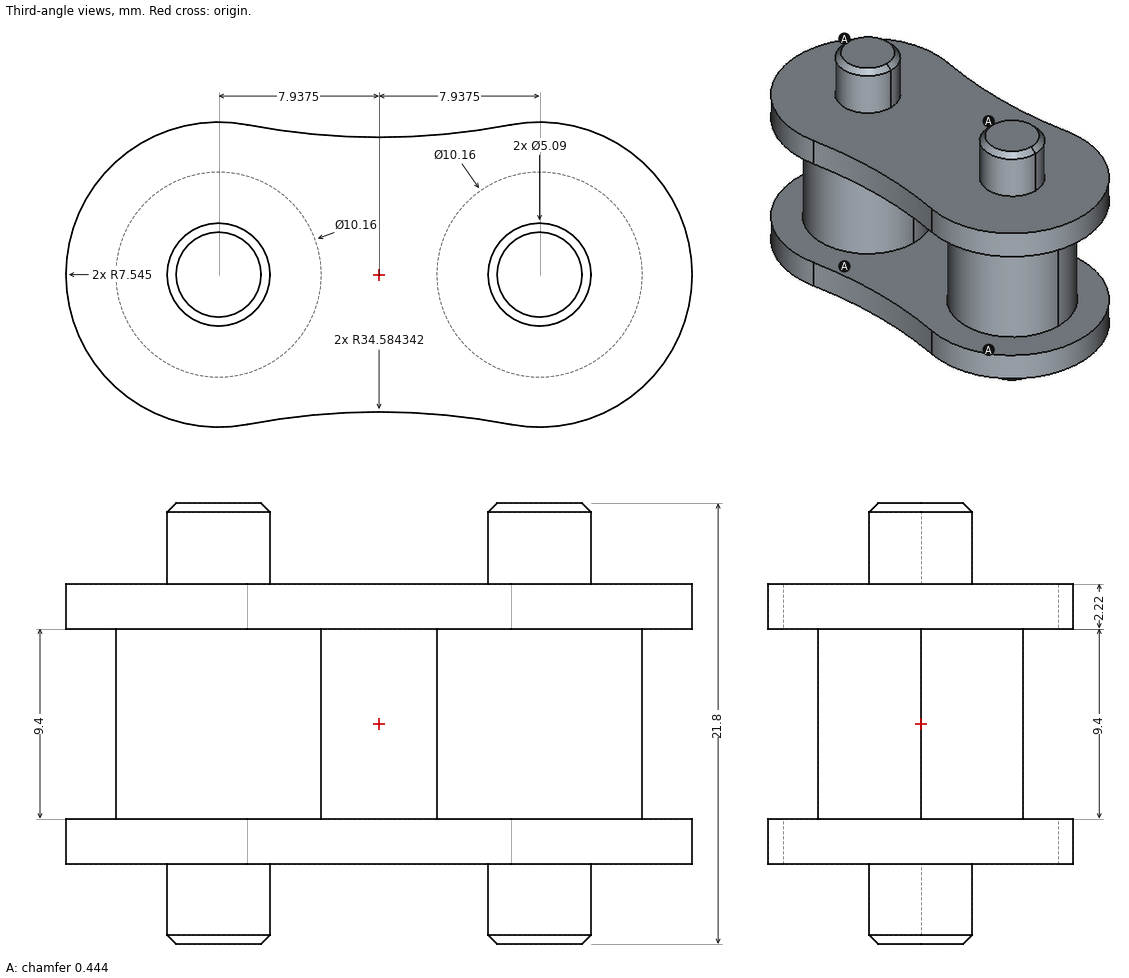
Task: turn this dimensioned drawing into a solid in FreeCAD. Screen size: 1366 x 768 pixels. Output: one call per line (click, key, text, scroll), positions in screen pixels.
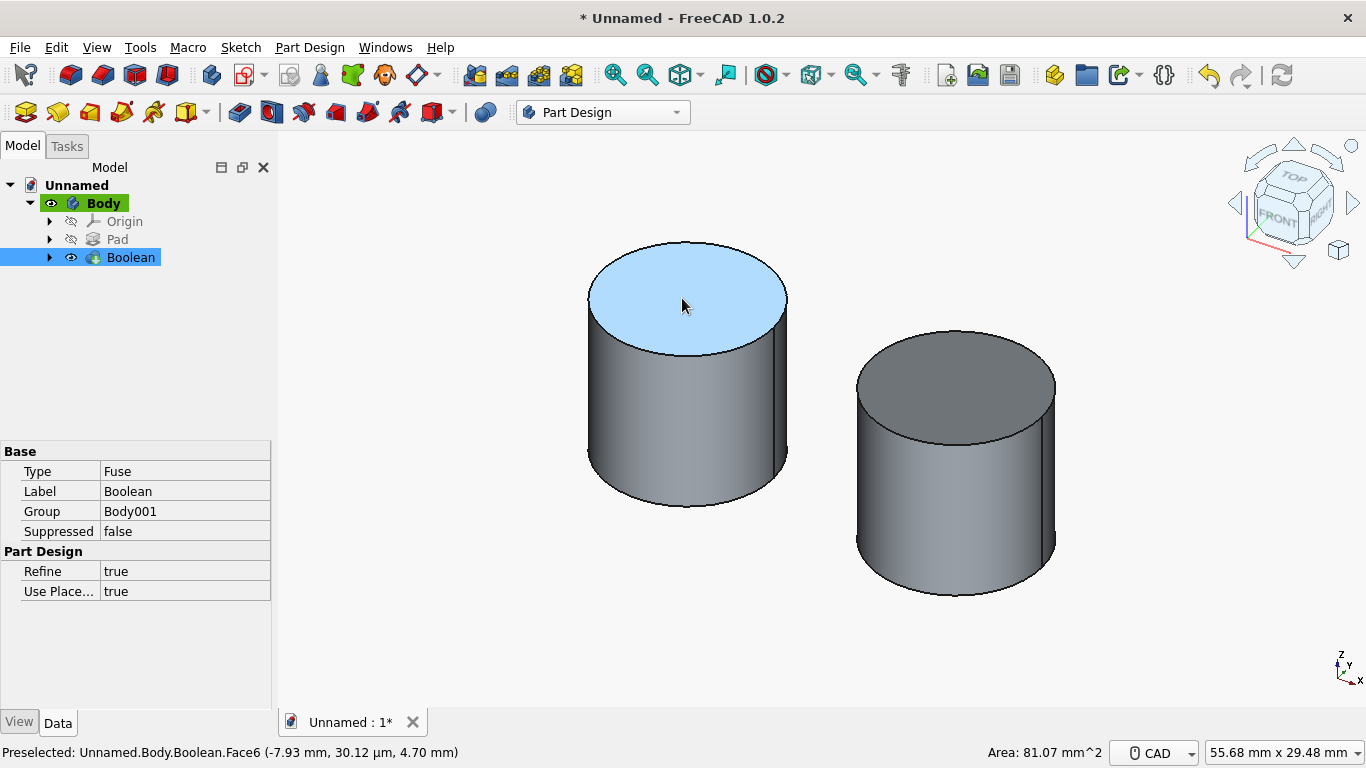
click(244, 76)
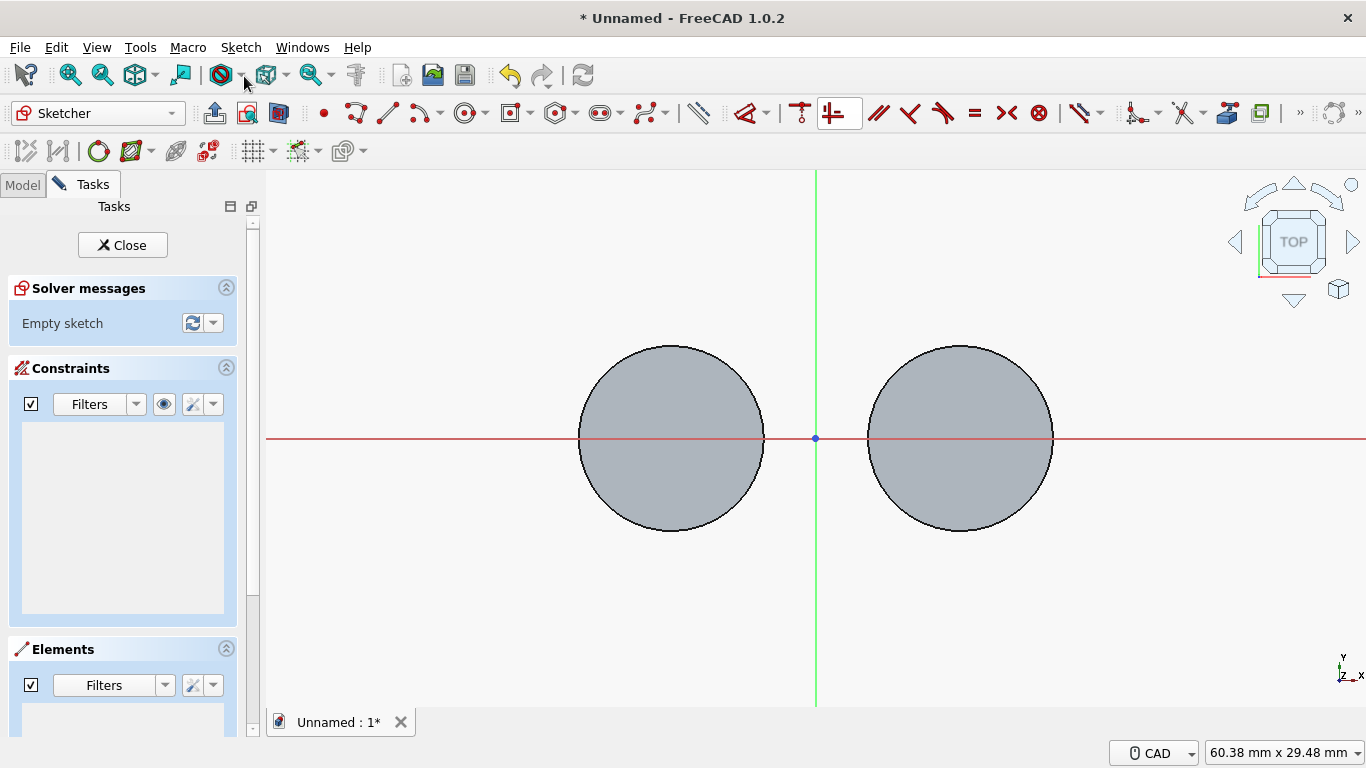
key(g)
key(3)
key(a)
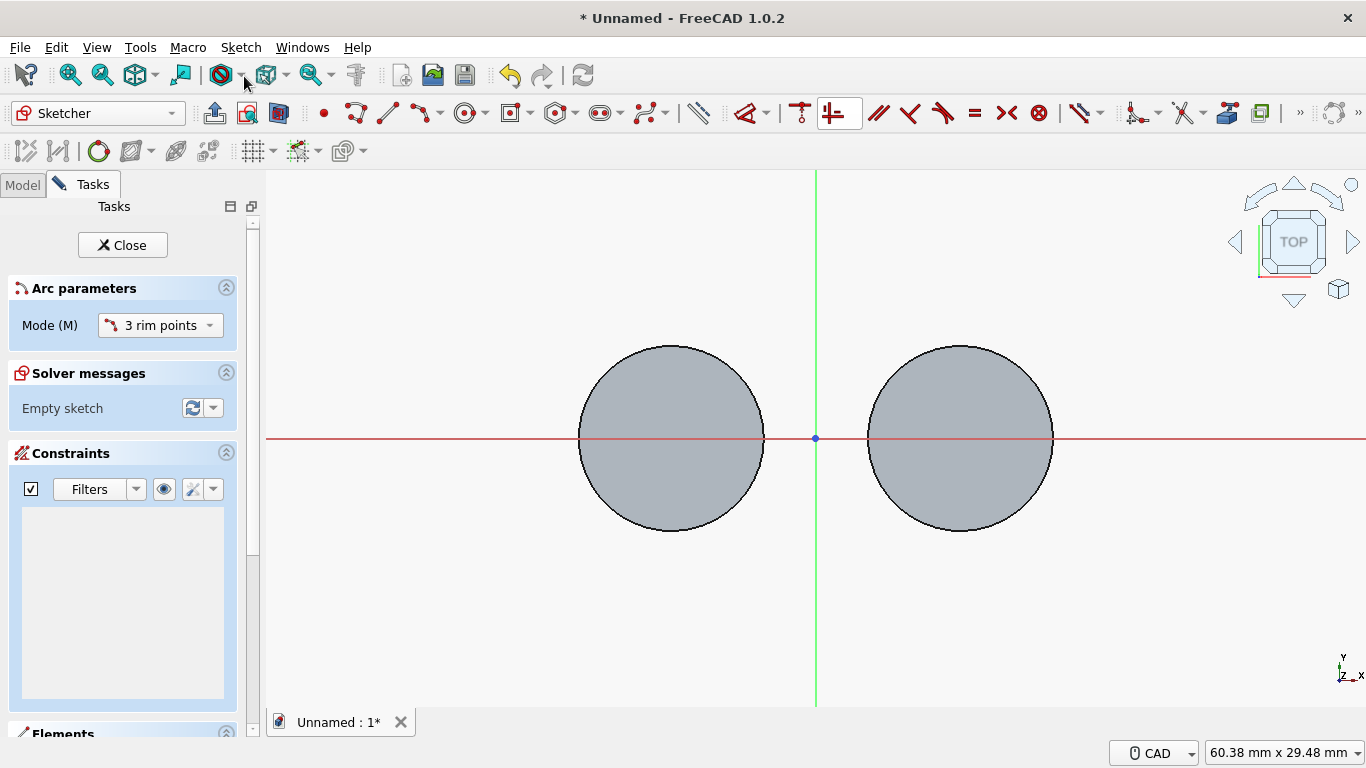
click(697, 304)
click(697, 573)
click(542, 391)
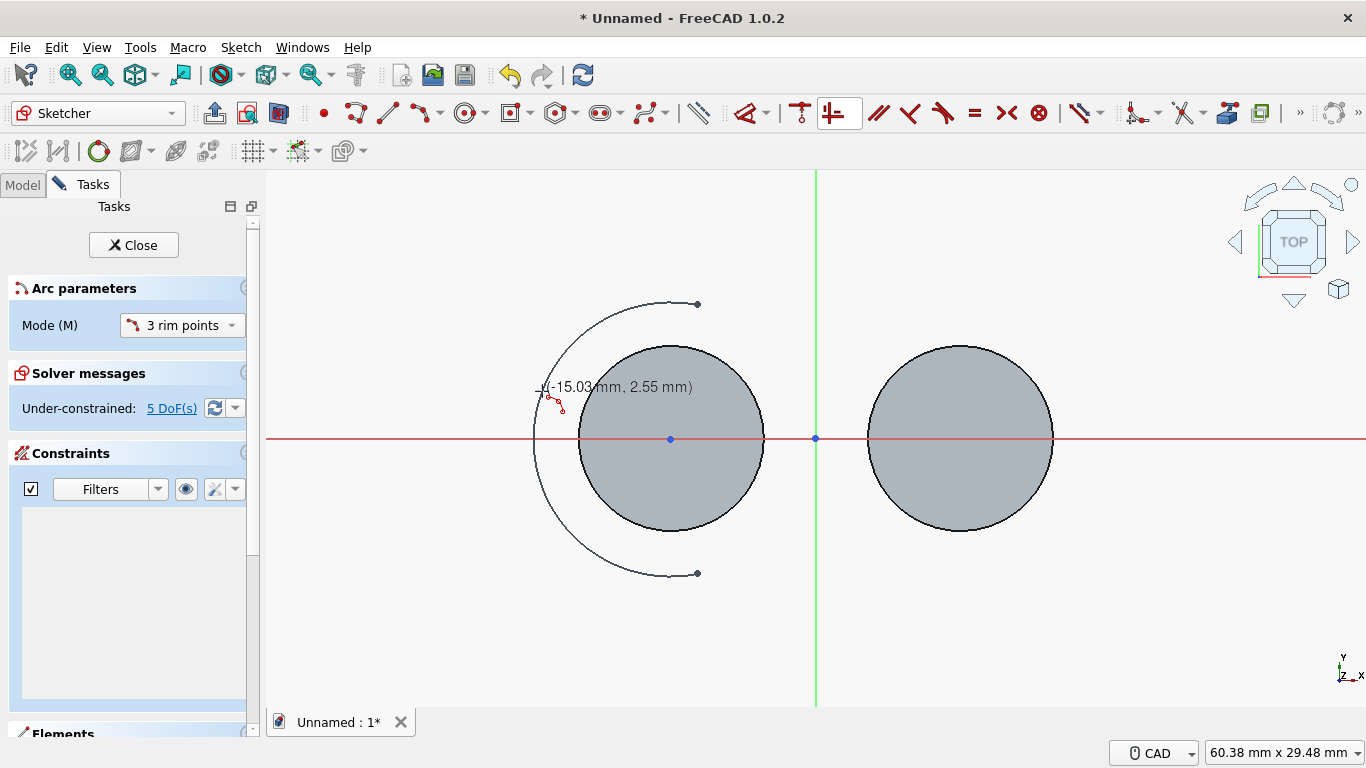
click(697, 574)
click(935, 573)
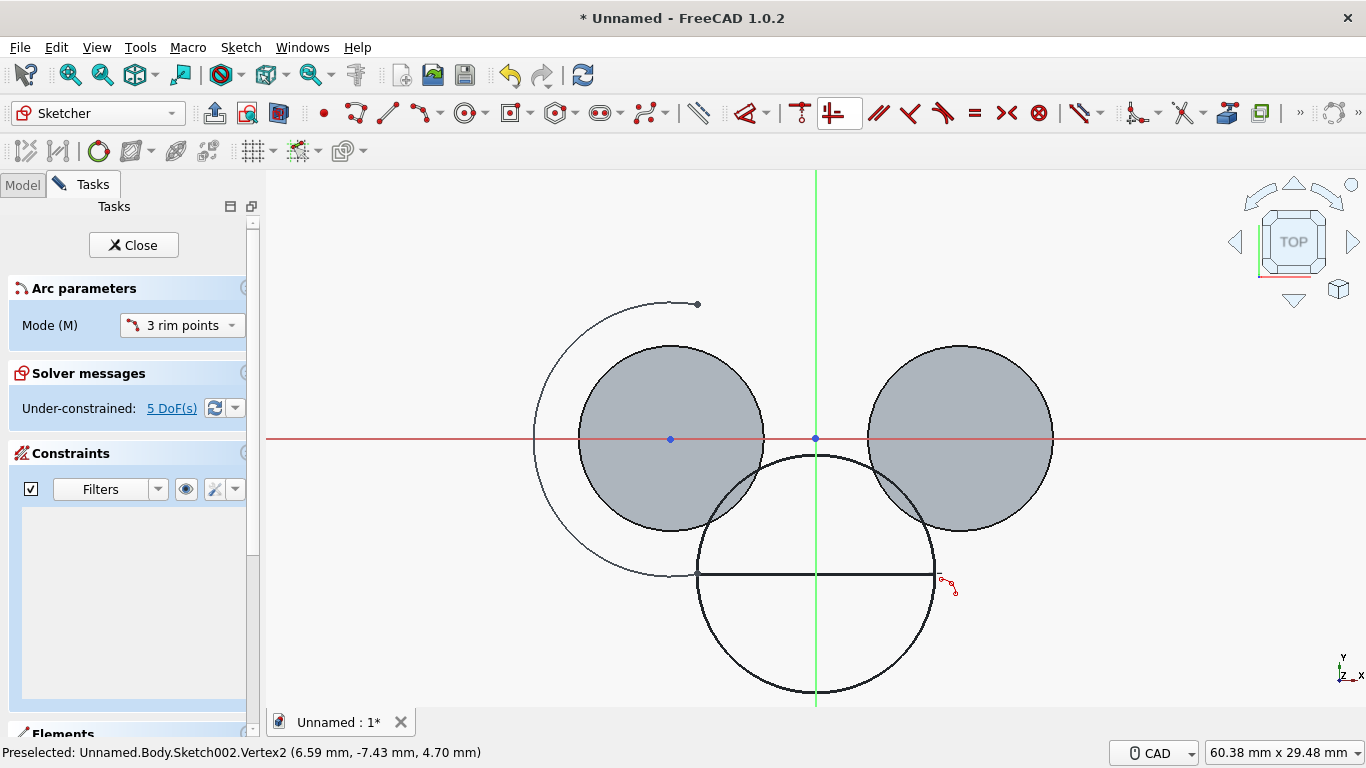
scroll(840, 563, up, 2)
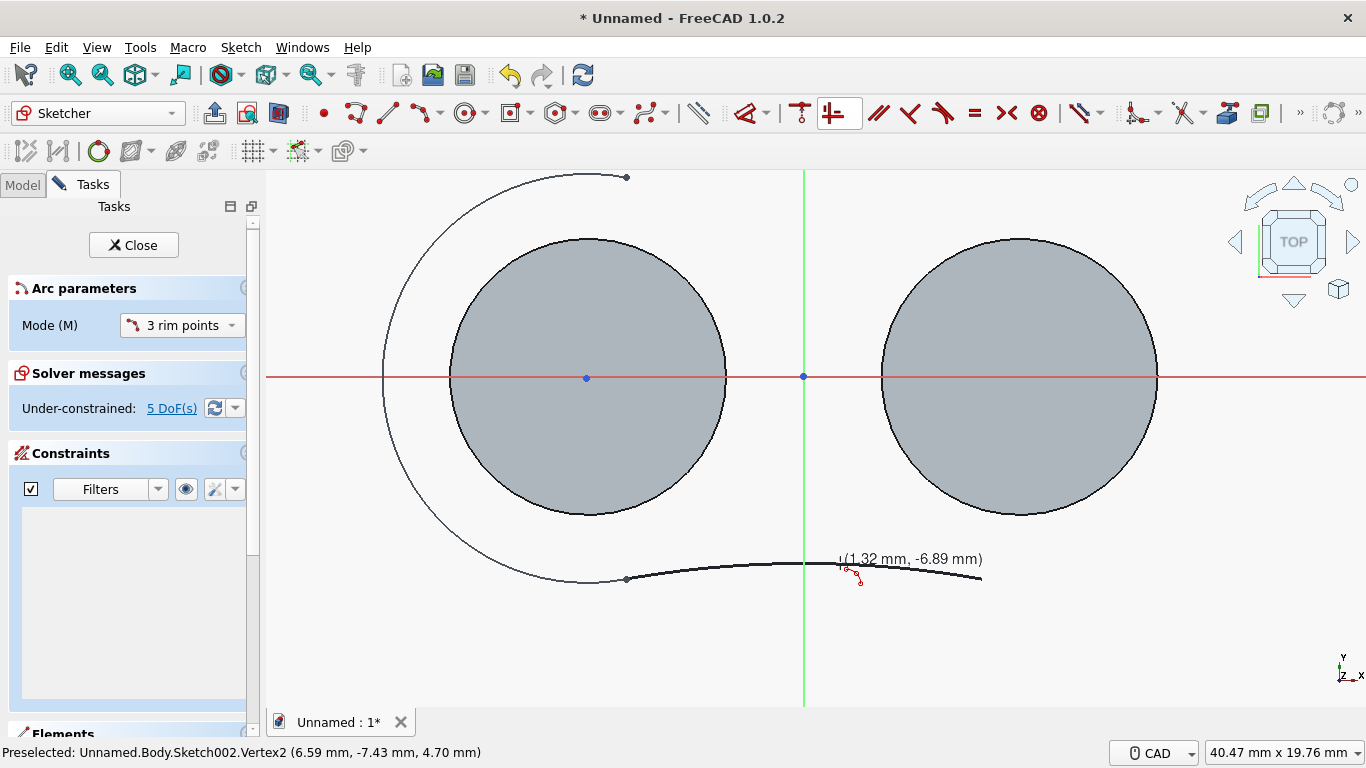
click(839, 562)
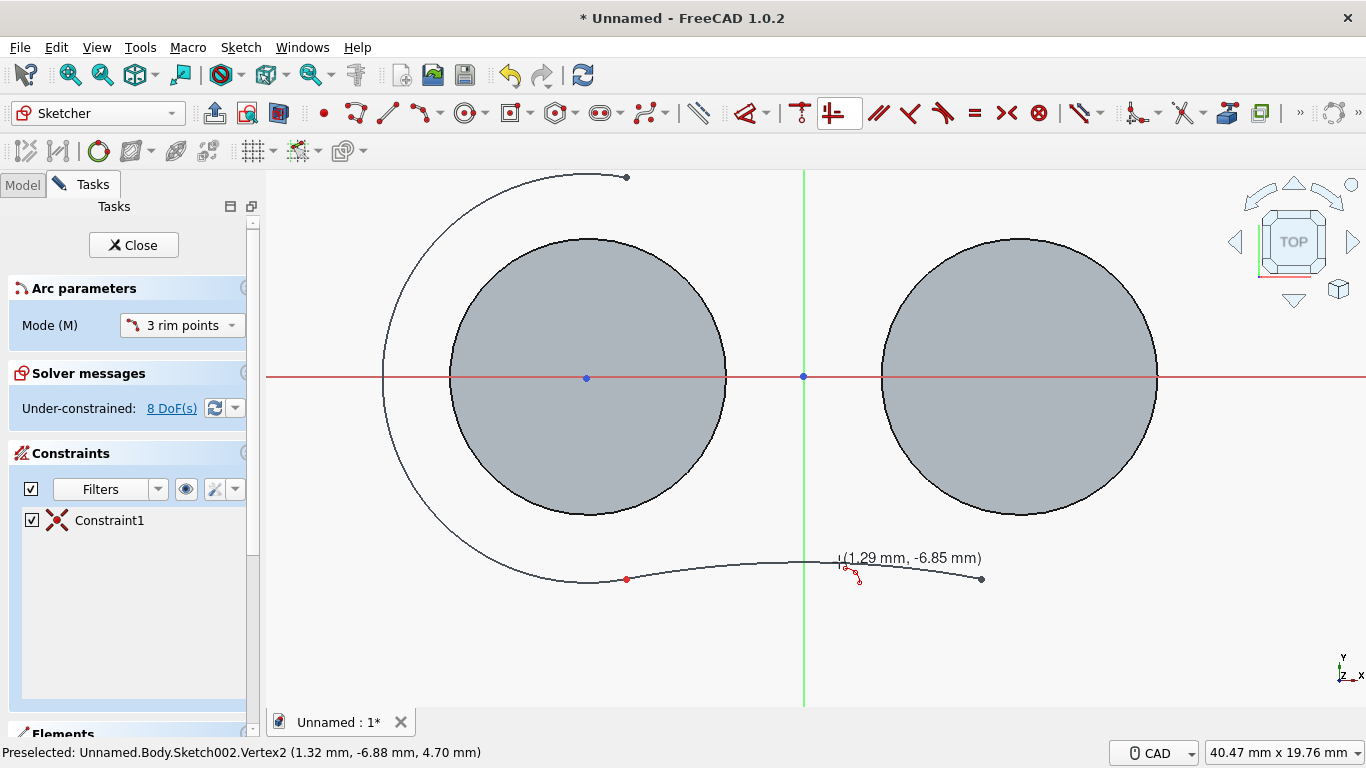
click(981, 579)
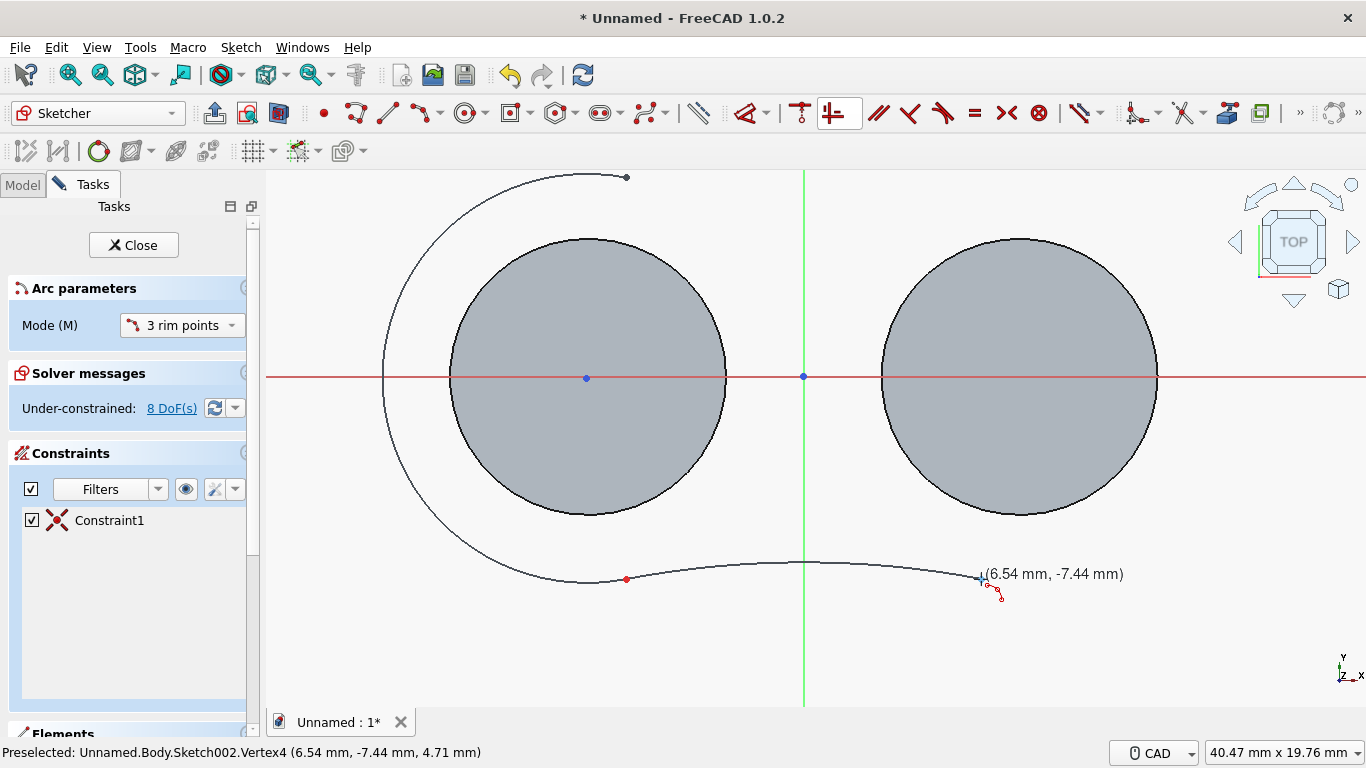
scroll(493, 679, down, 1)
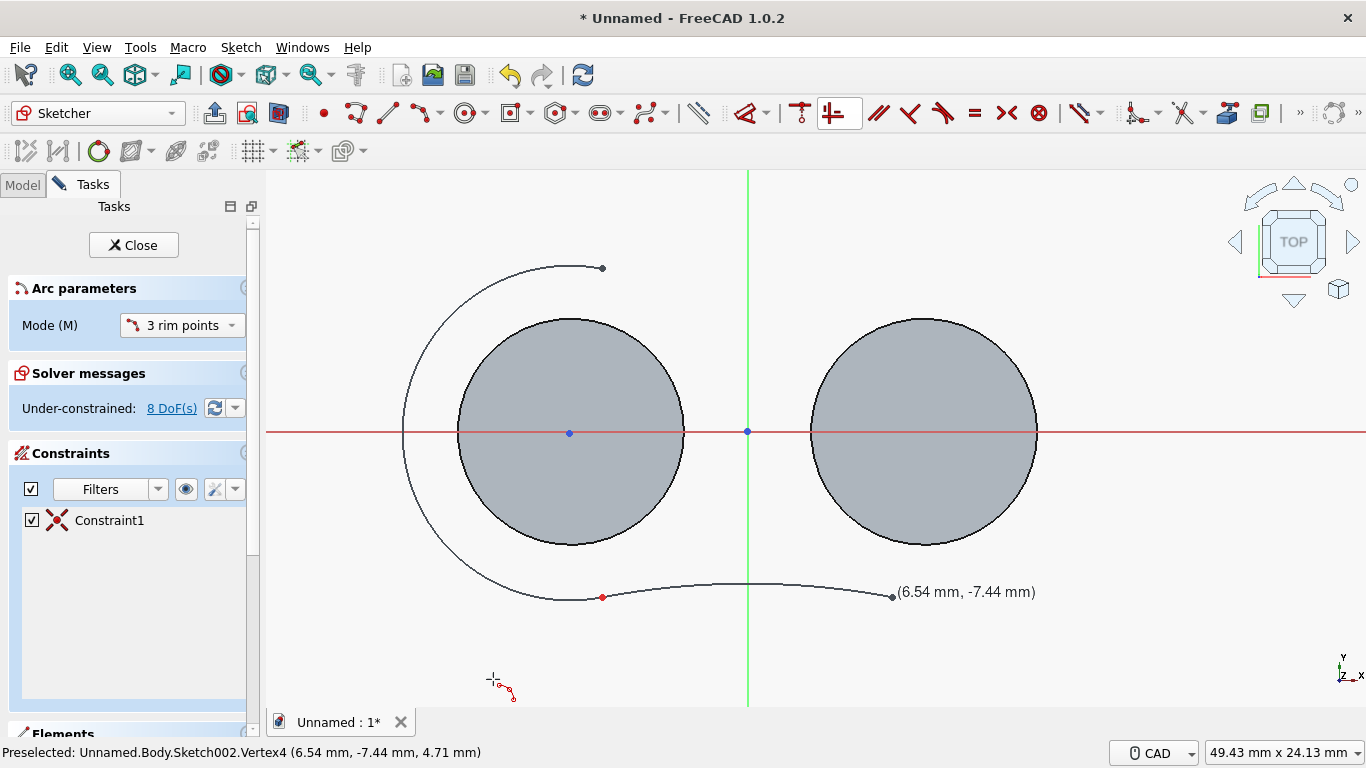
click(892, 267)
click(1082, 490)